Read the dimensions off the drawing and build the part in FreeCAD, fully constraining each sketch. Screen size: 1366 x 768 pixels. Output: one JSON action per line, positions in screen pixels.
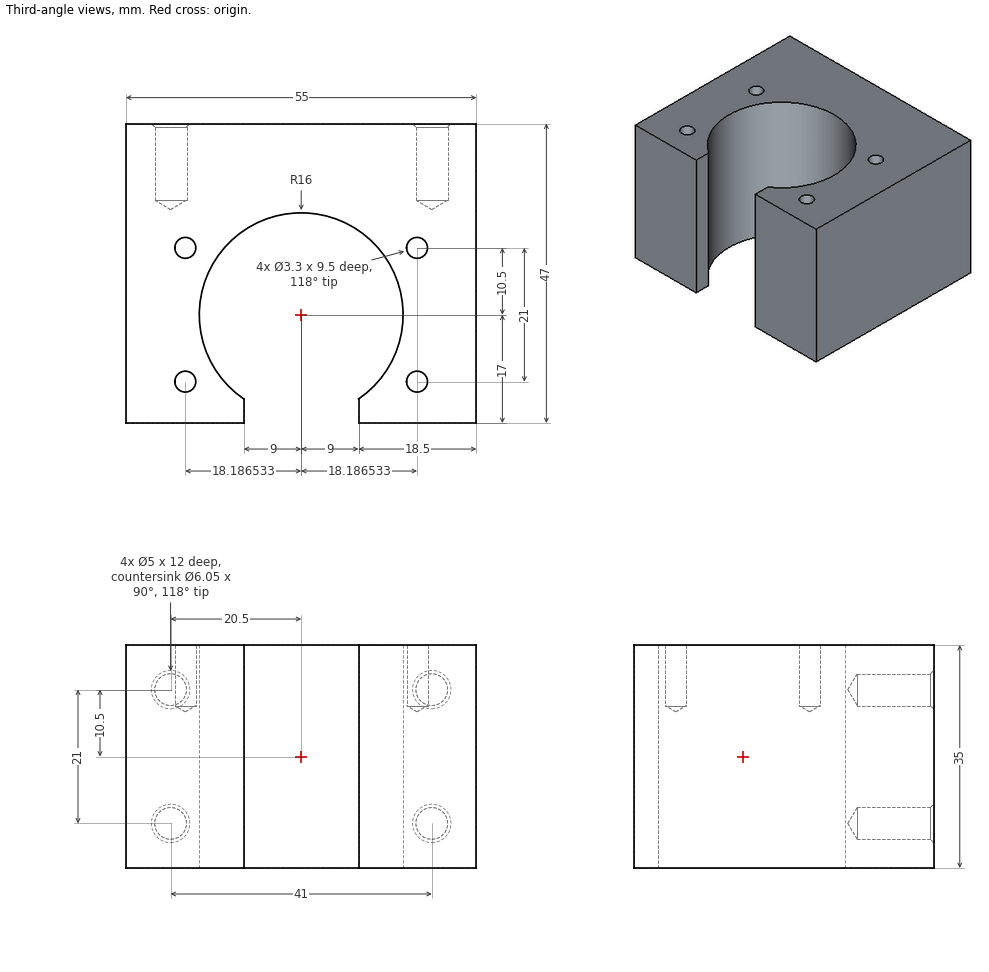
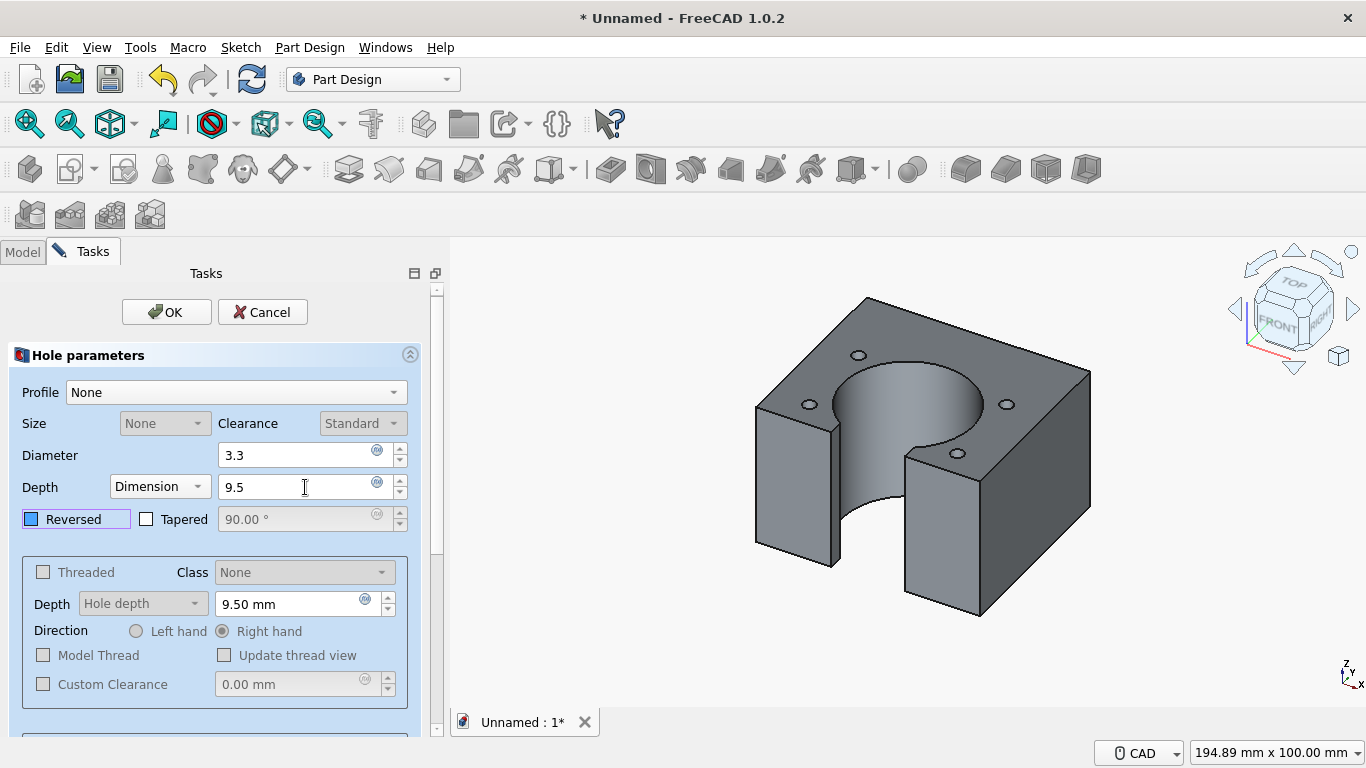
{"action": "left_click", "coordinate": [167, 312]}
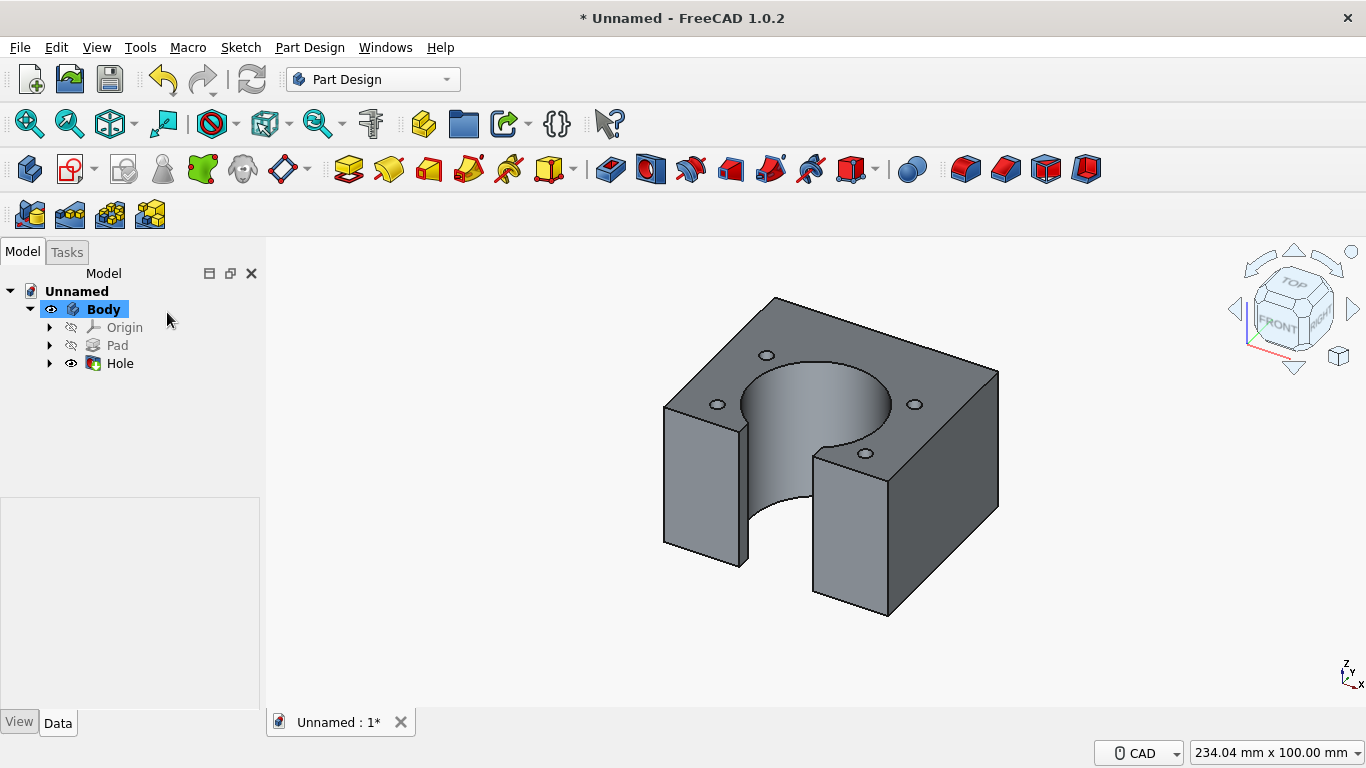
{"action": "key", "text": "4"}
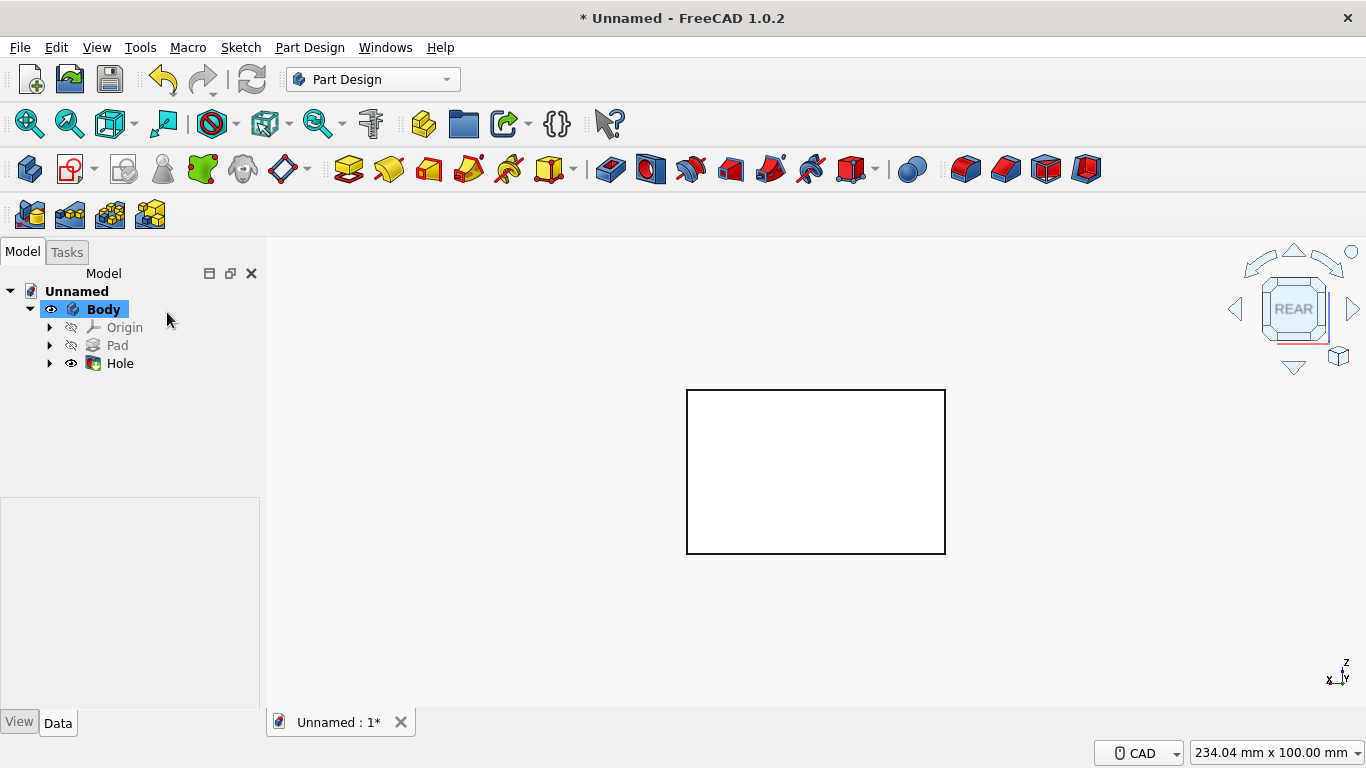
{"action": "left_click", "coordinate": [30, 124]}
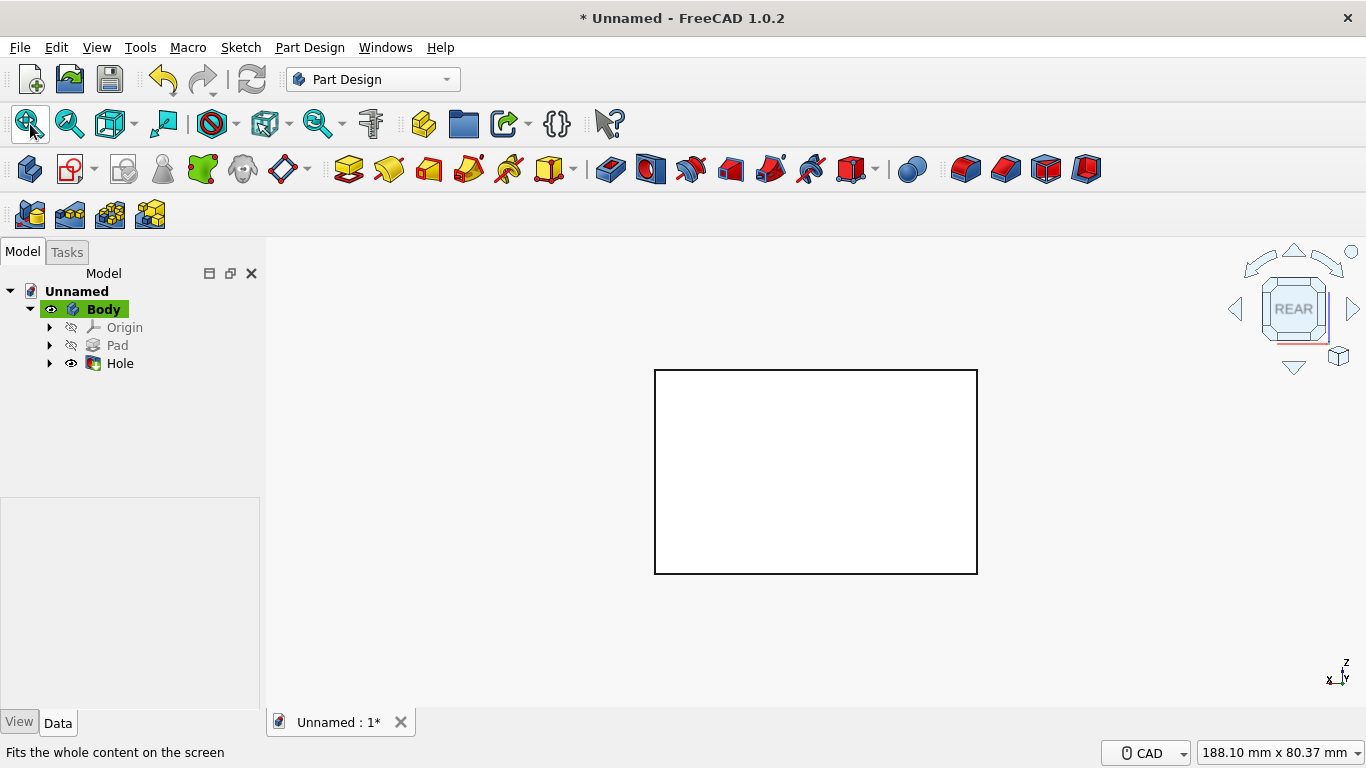
{"action": "left_click", "coordinate": [770, 471]}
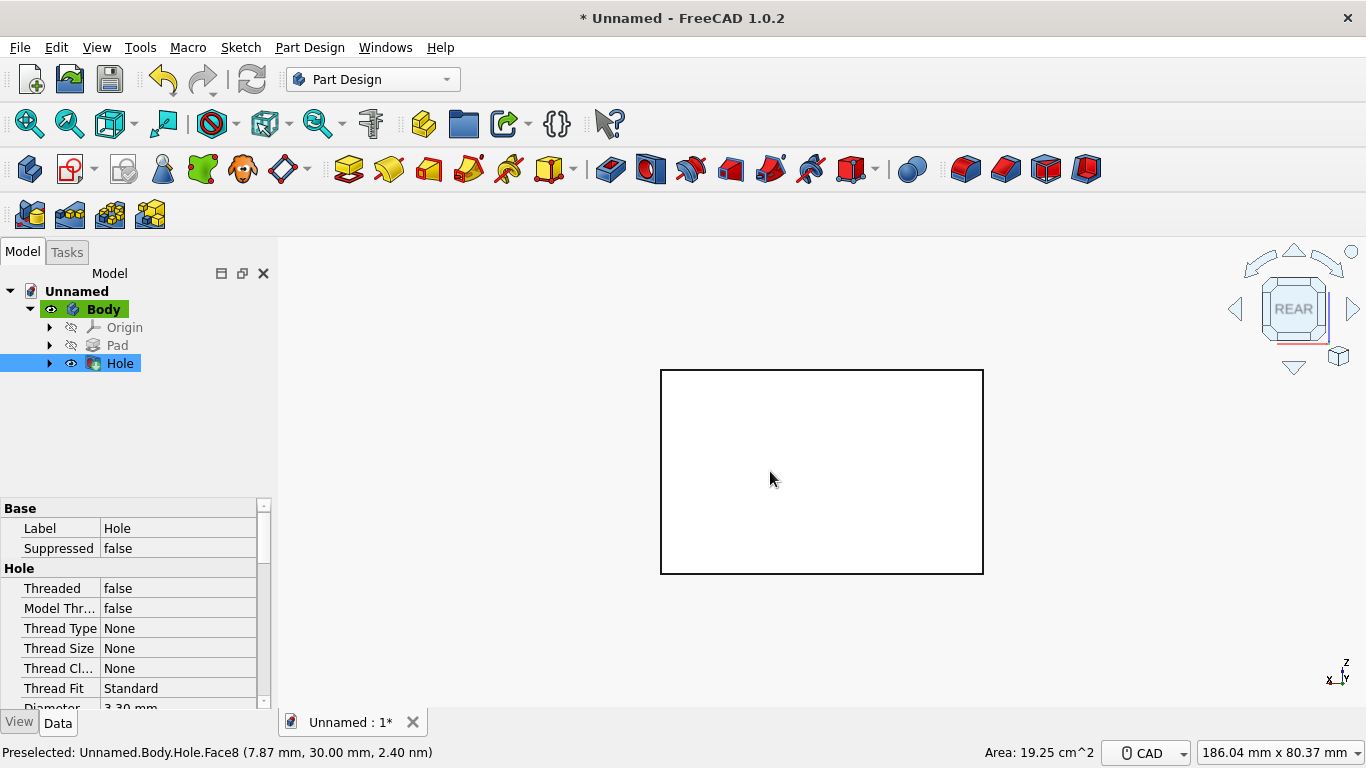
{"action": "left_click", "coordinate": [70, 170]}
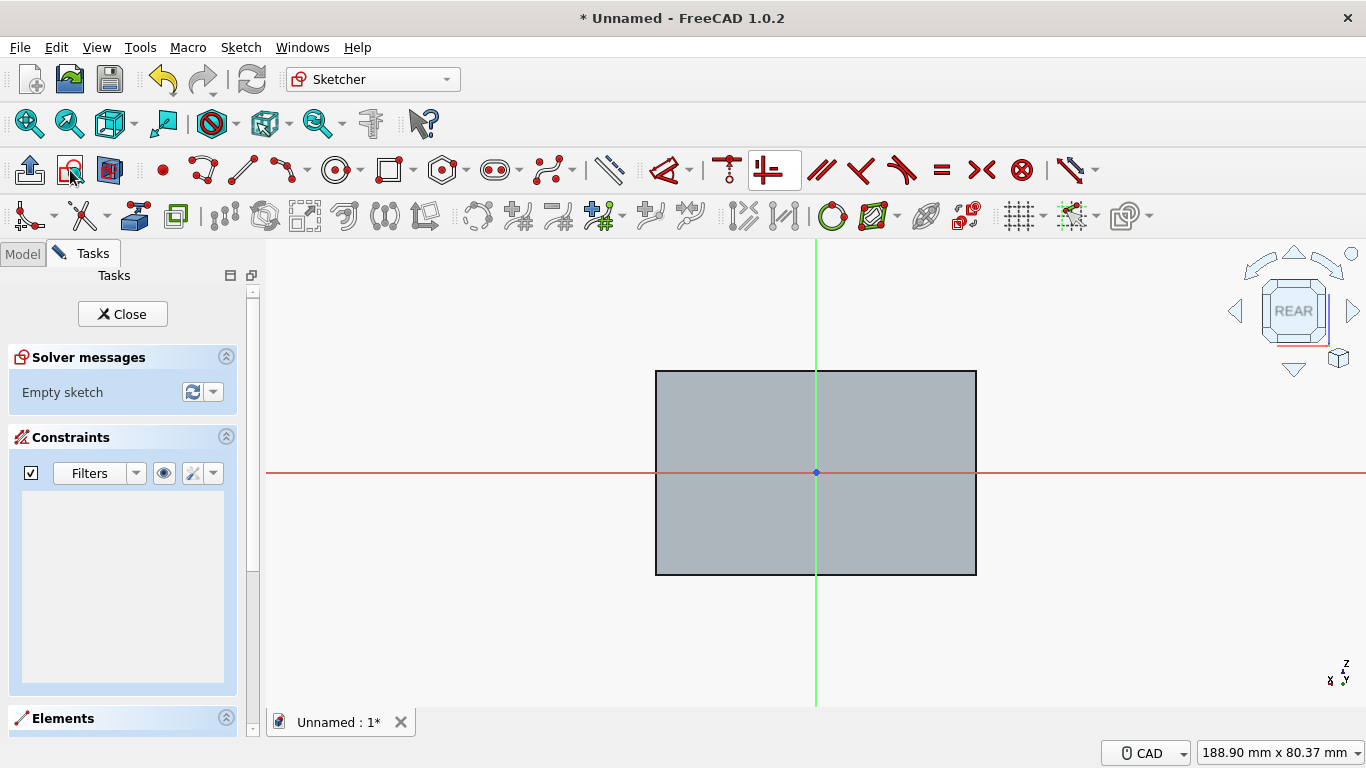
{"action": "scroll", "coordinate": [899, 473], "scroll_direction": "up", "scroll_amount": 3}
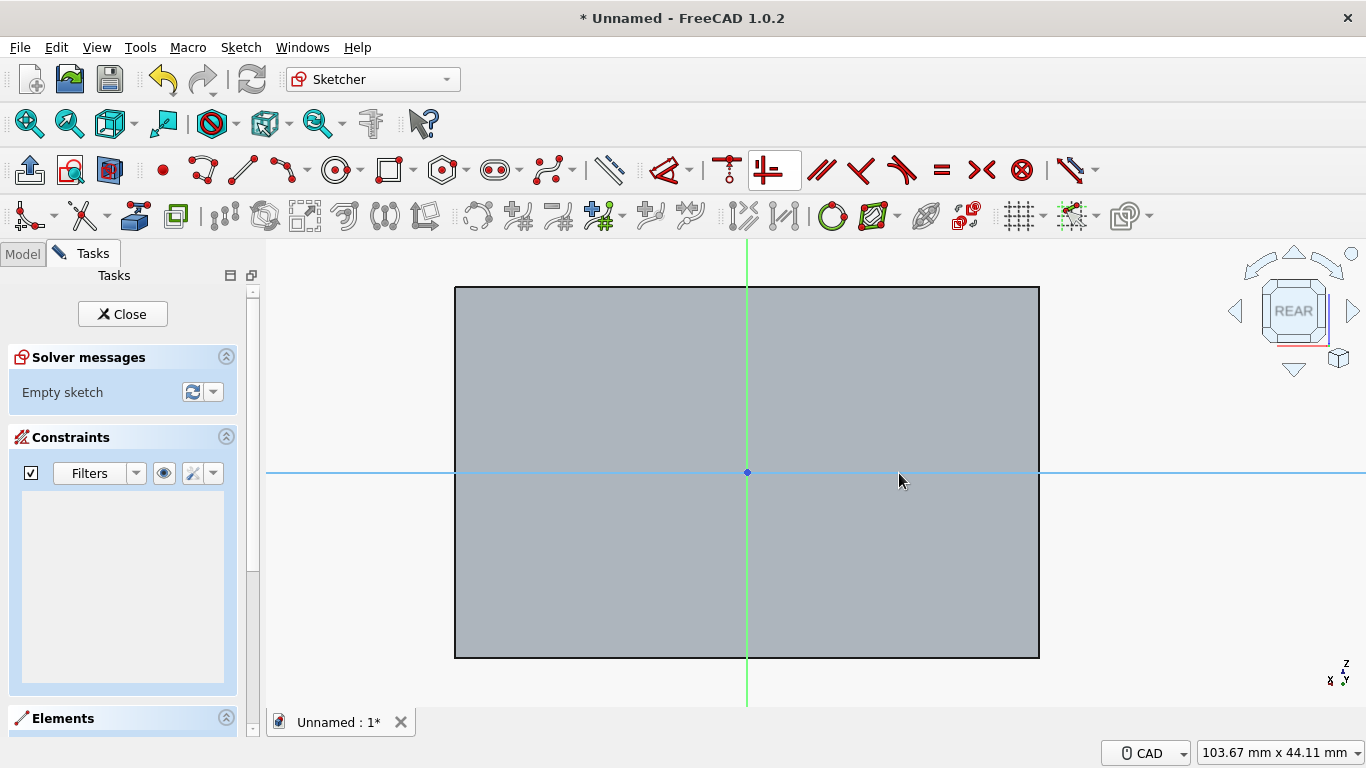
{"action": "left_click", "coordinate": [336, 170]}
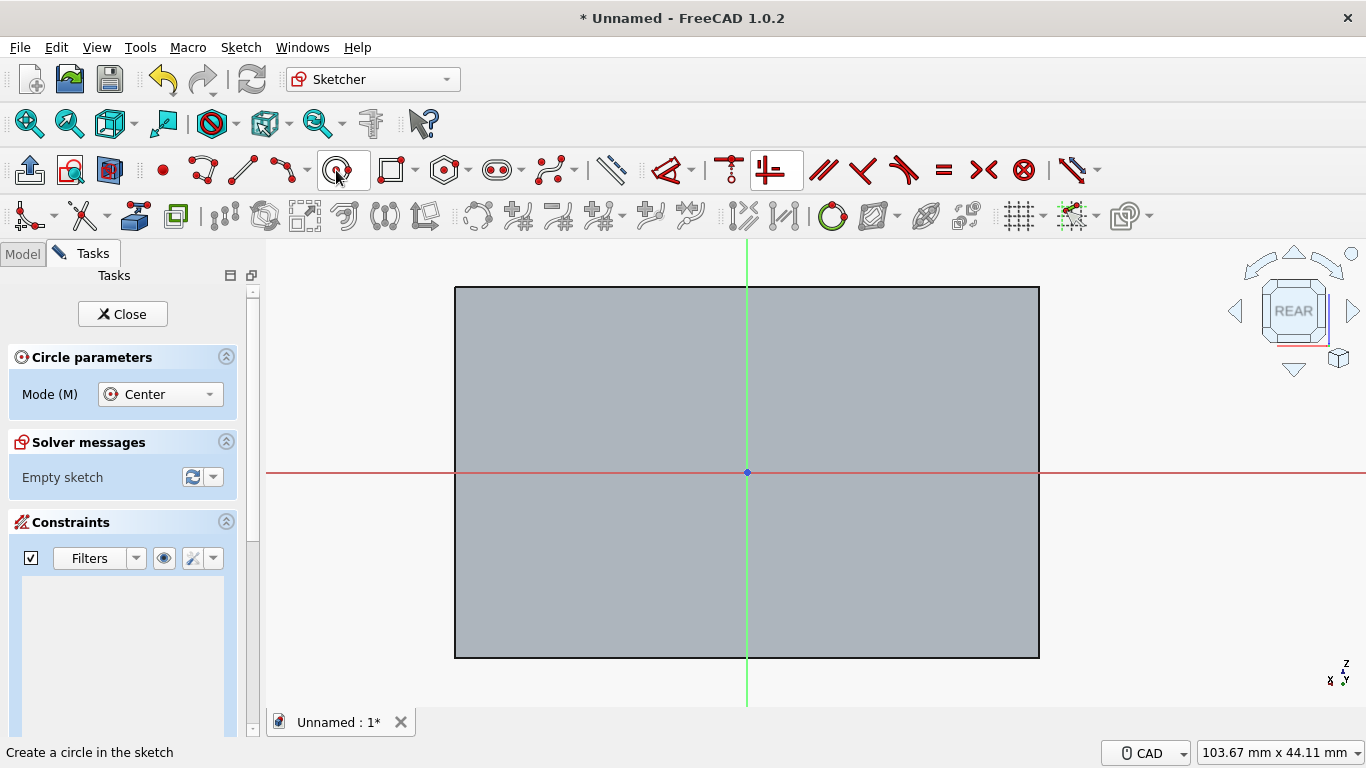
{"action": "left_click", "coordinate": [965, 361]}
{"action": "mouse_move", "coordinate": [984, 342]}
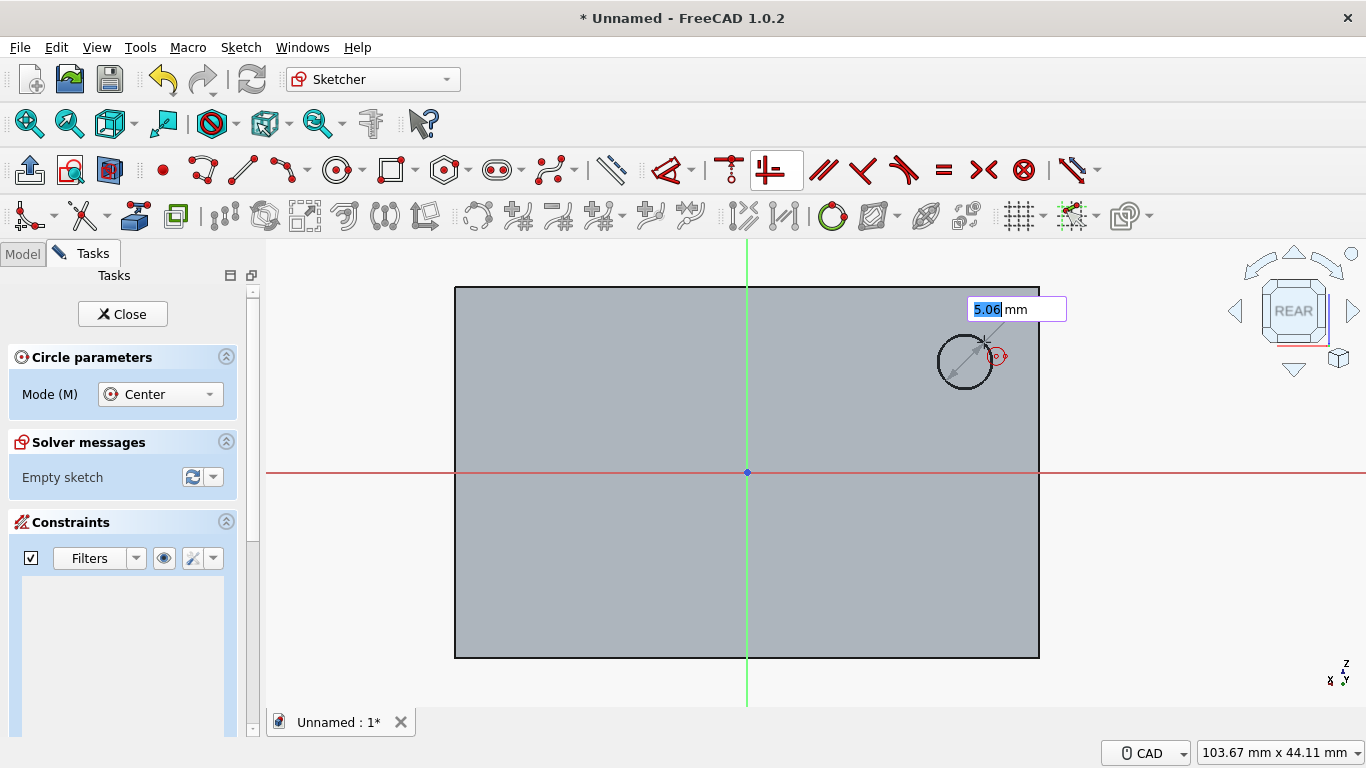
{"action": "type", "text": "5"}
{"action": "key", "text": "Return"}